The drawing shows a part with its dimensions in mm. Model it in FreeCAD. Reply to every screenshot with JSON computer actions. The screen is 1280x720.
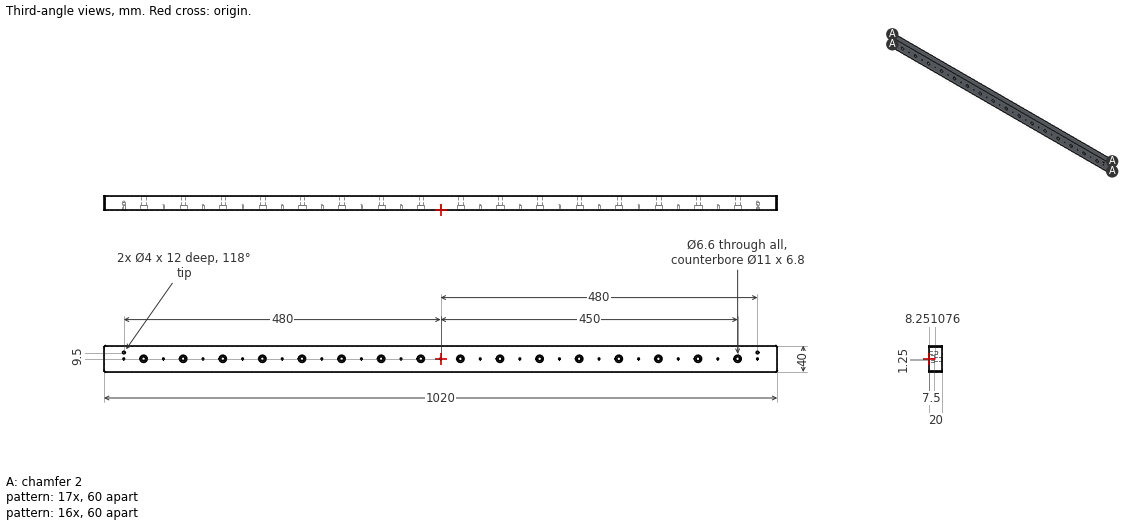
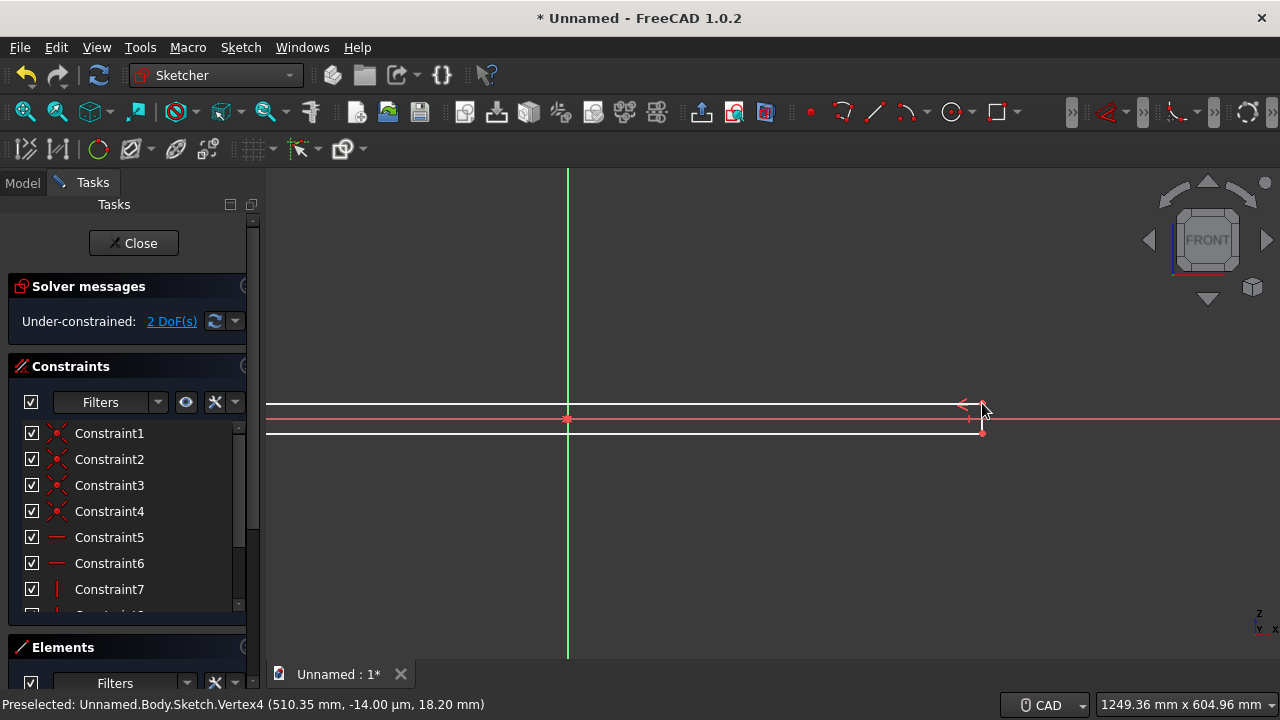
{"action": "left_click", "coordinate": [1106, 112]}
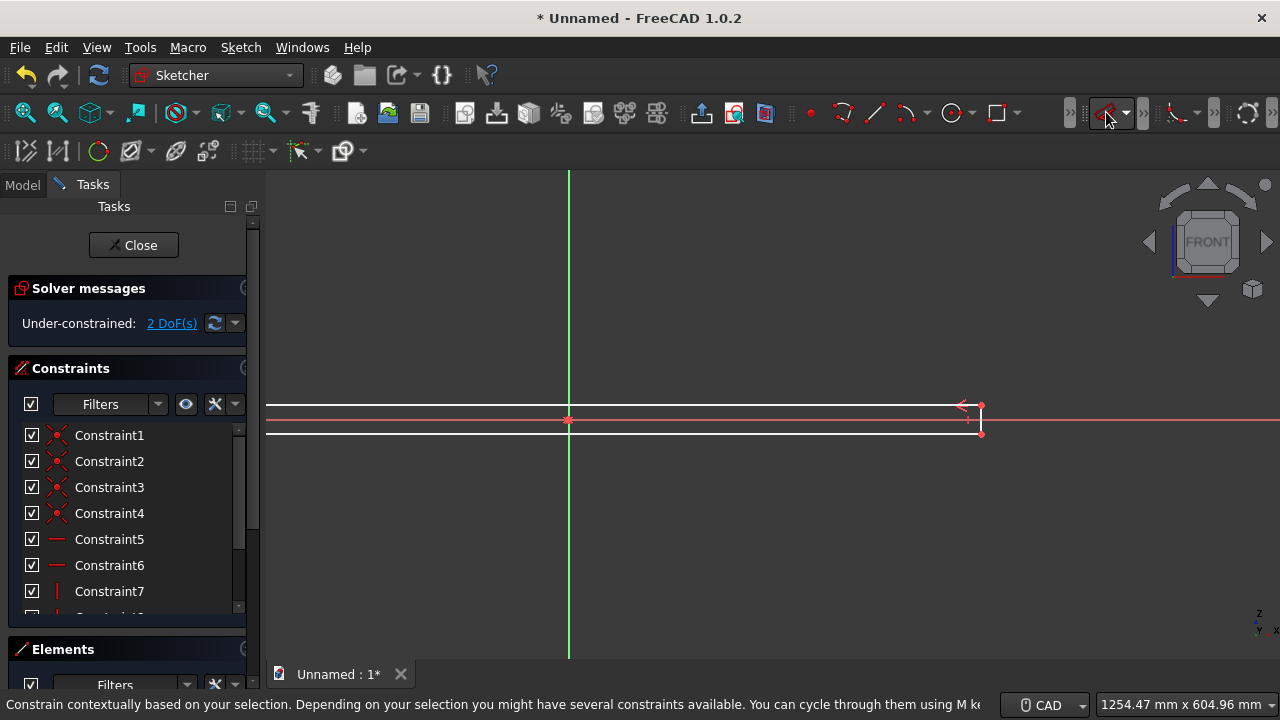
{"action": "scroll", "coordinate": [981, 423], "scroll_direction": "up", "scroll_amount": 2}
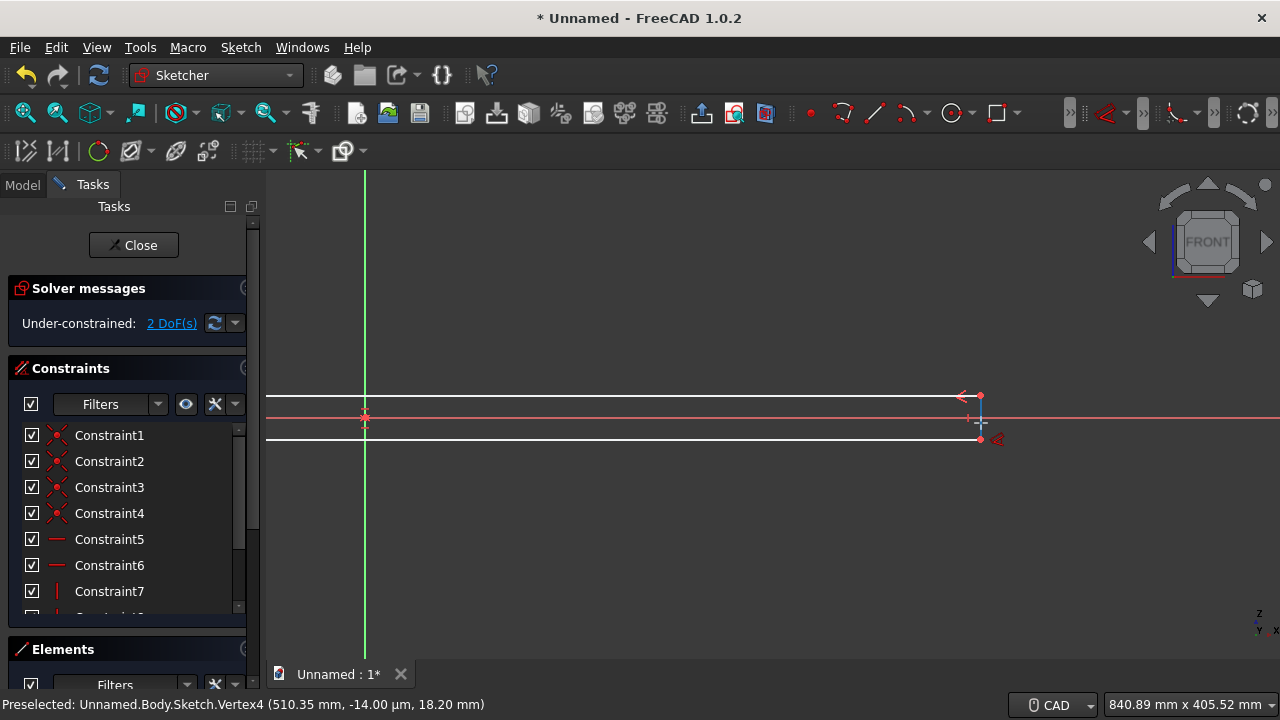
{"action": "left_click", "coordinate": [981, 422]}
{"action": "left_click", "coordinate": [1015, 403]}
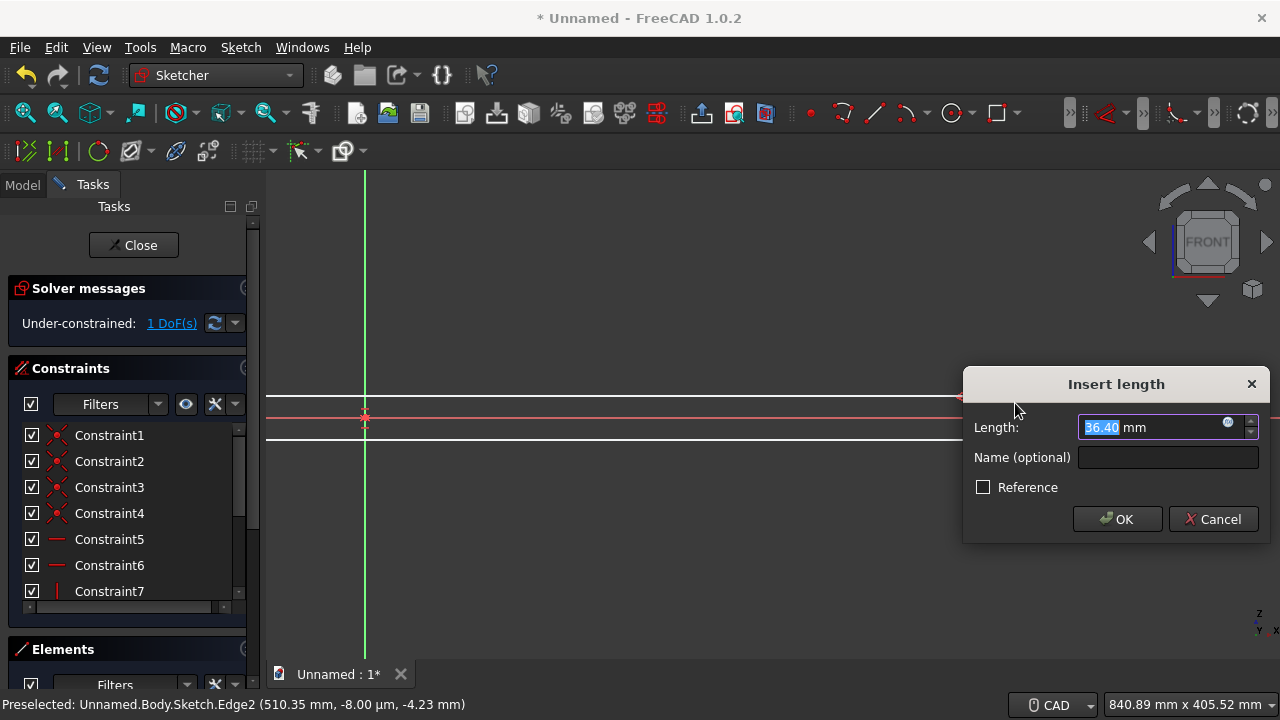
{"action": "type", "text": "40"}
{"action": "key", "text": "Return"}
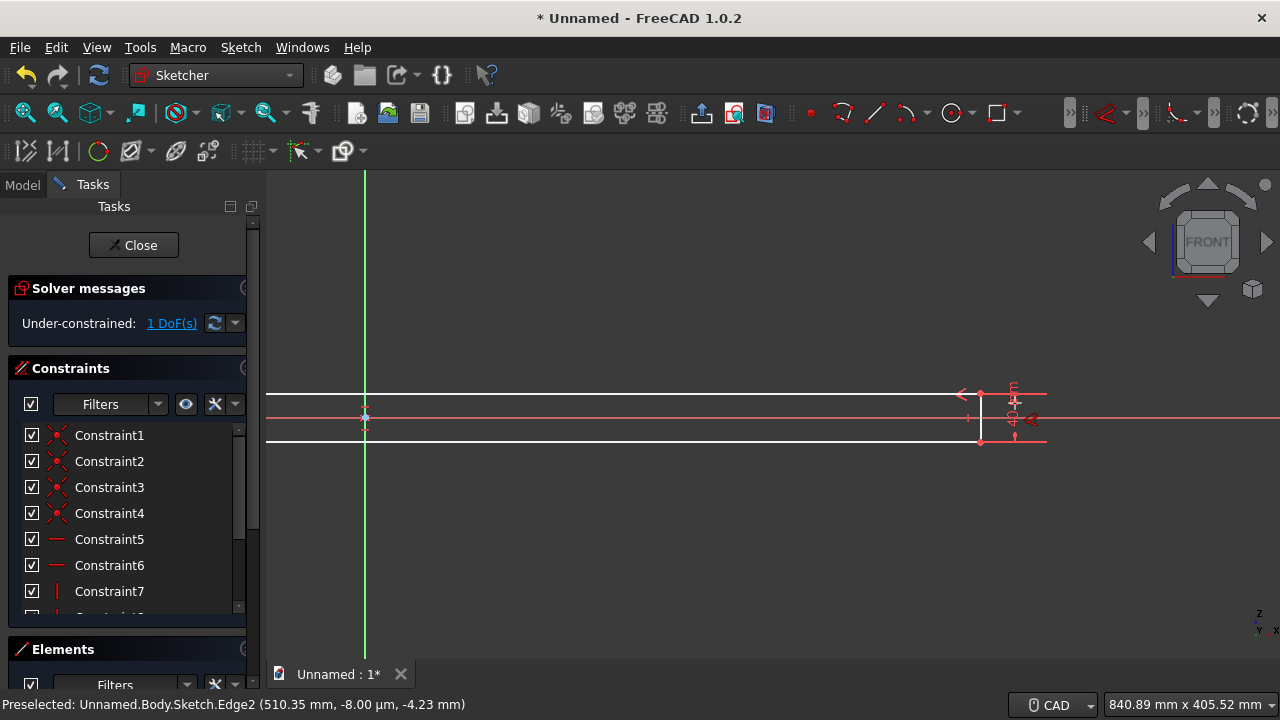
{"action": "left_click", "coordinate": [612, 442]}
{"action": "left_click", "coordinate": [637, 476]}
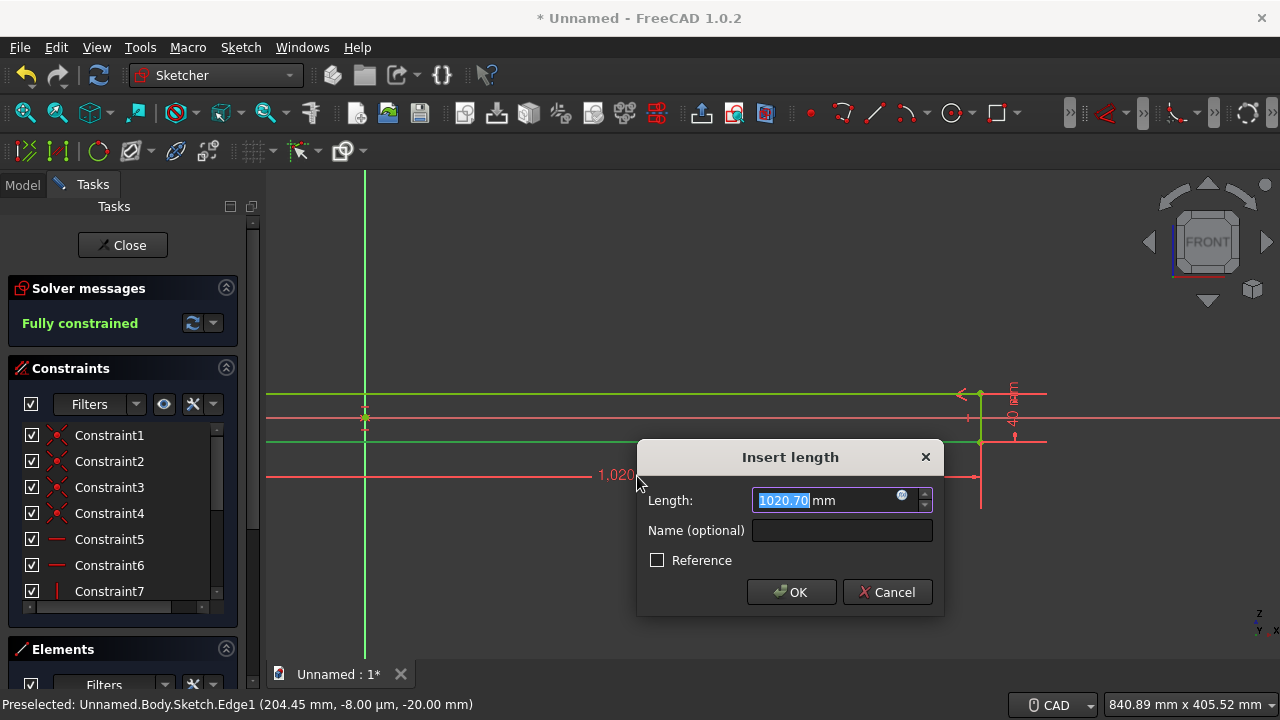
{"action": "type", "text": "1020"}
{"action": "key", "text": "Return"}
{"action": "key", "text": "Escape"}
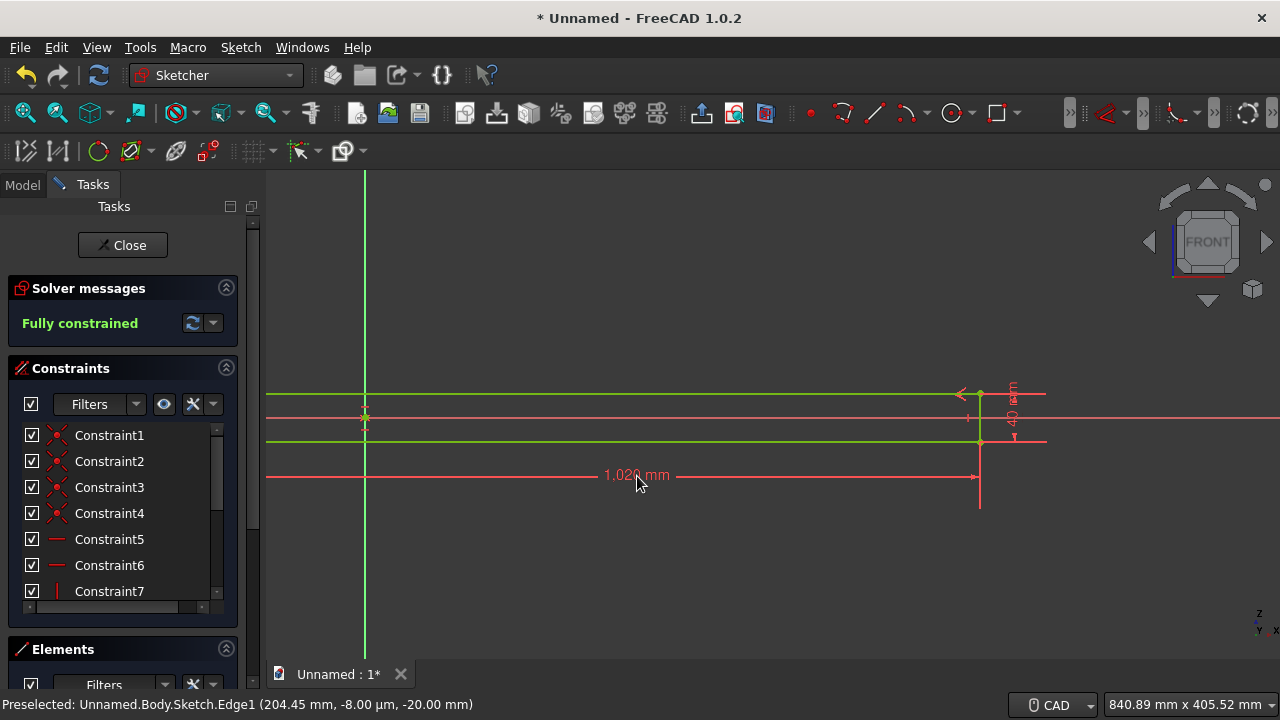
{"action": "left_click", "coordinate": [123, 245]}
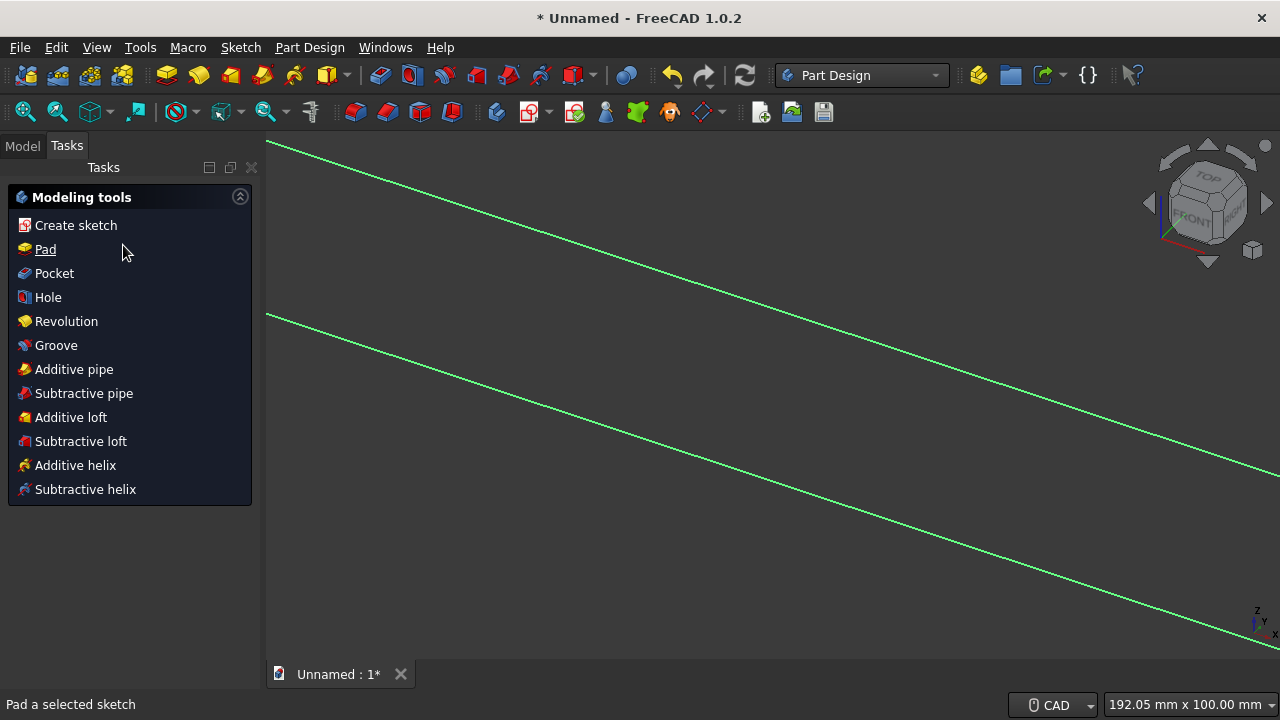
{"action": "left_click", "coordinate": [168, 76]}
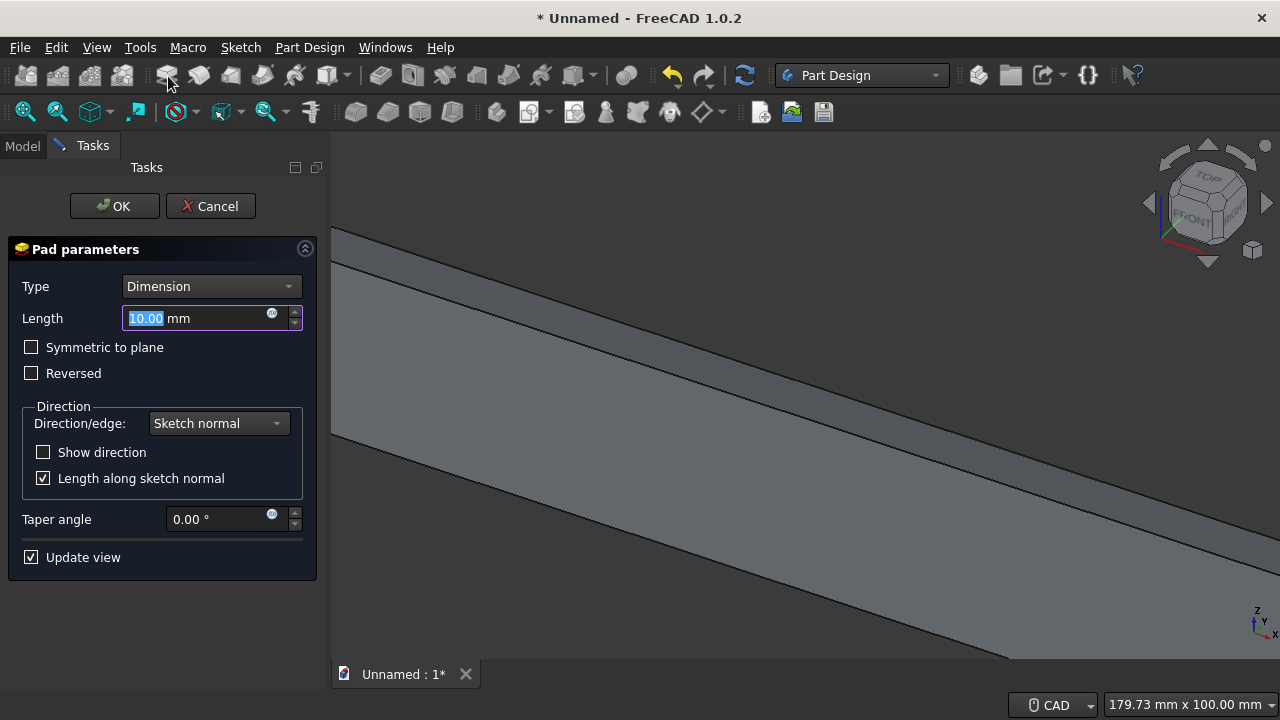
{"action": "type", "text": "20"}
{"action": "key", "text": "Tab"}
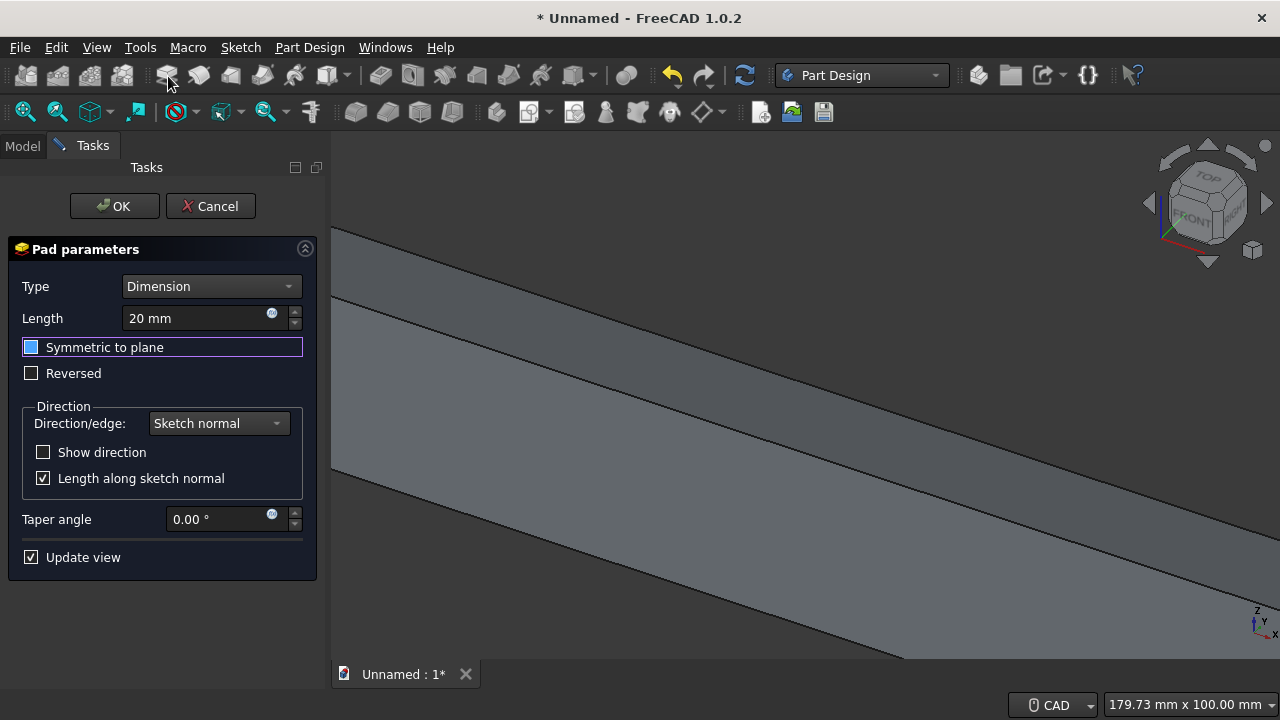
{"action": "left_click", "coordinate": [30, 373]}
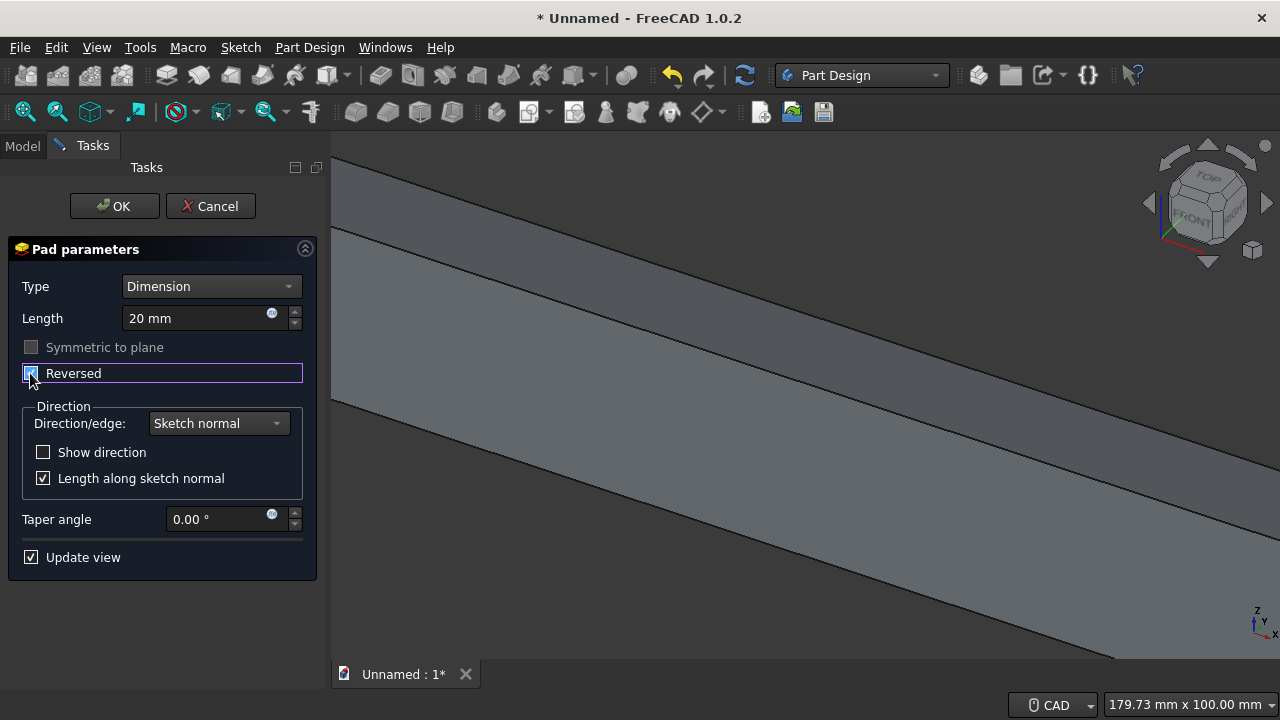
{"action": "left_click", "coordinate": [115, 206]}